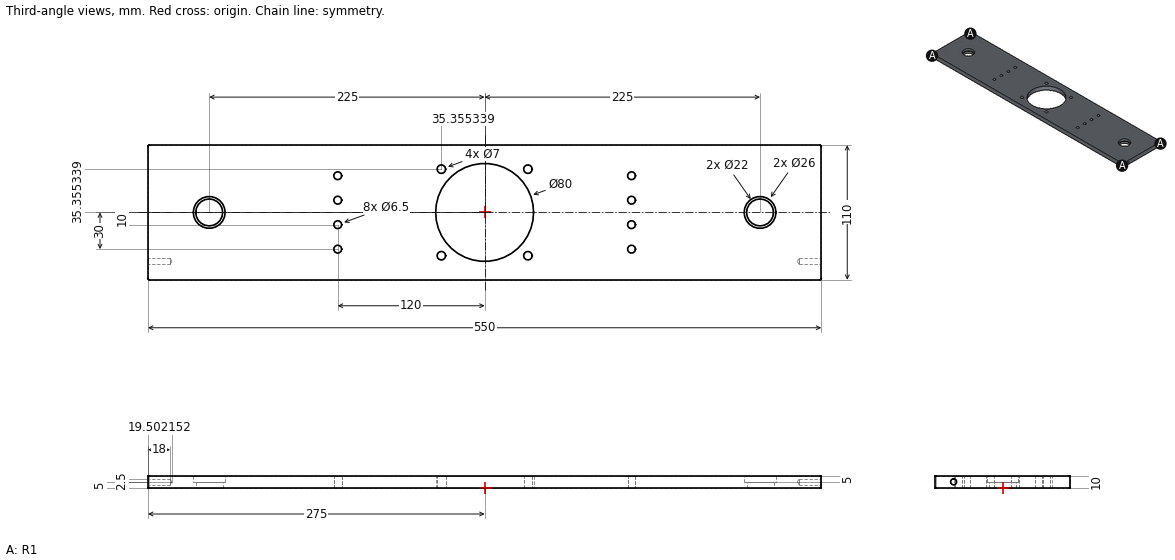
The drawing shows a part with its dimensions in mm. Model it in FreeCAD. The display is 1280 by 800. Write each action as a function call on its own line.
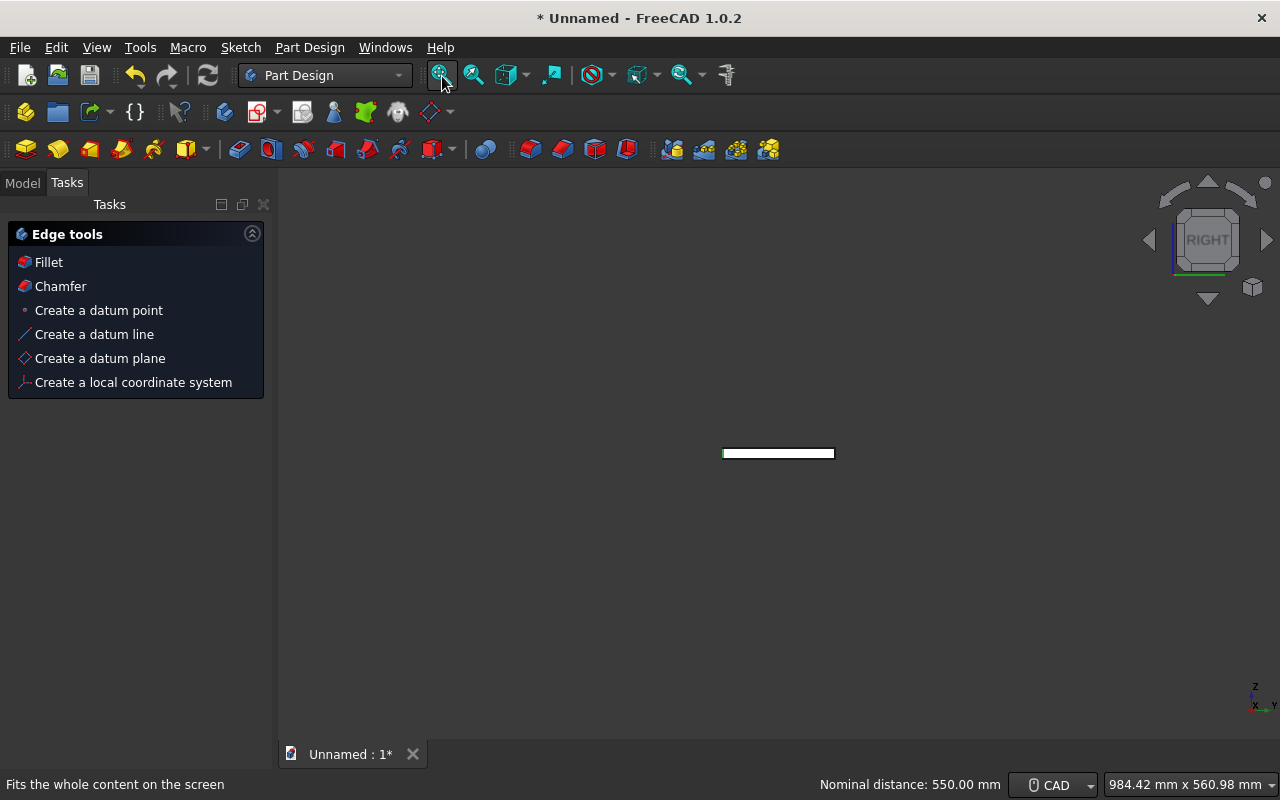
scroll(835, 452, up, 7)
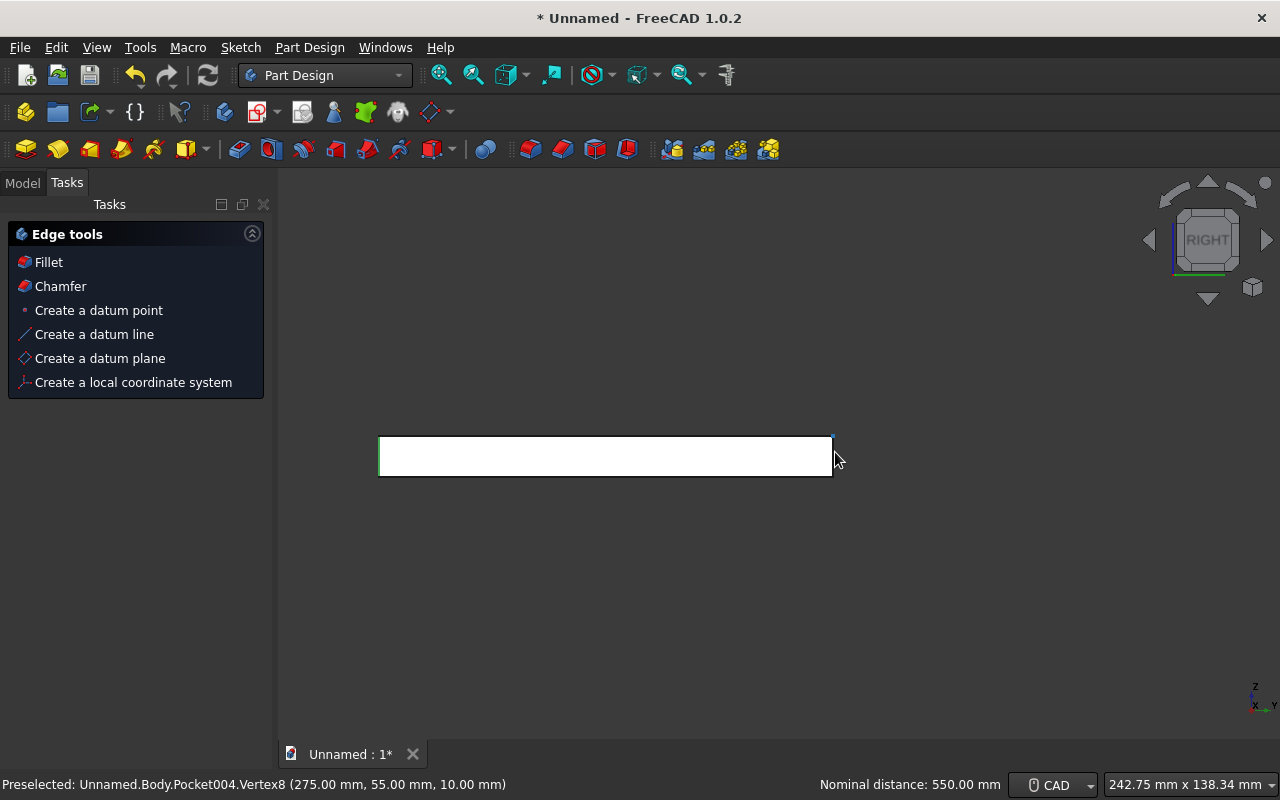
click(833, 456, ctrl)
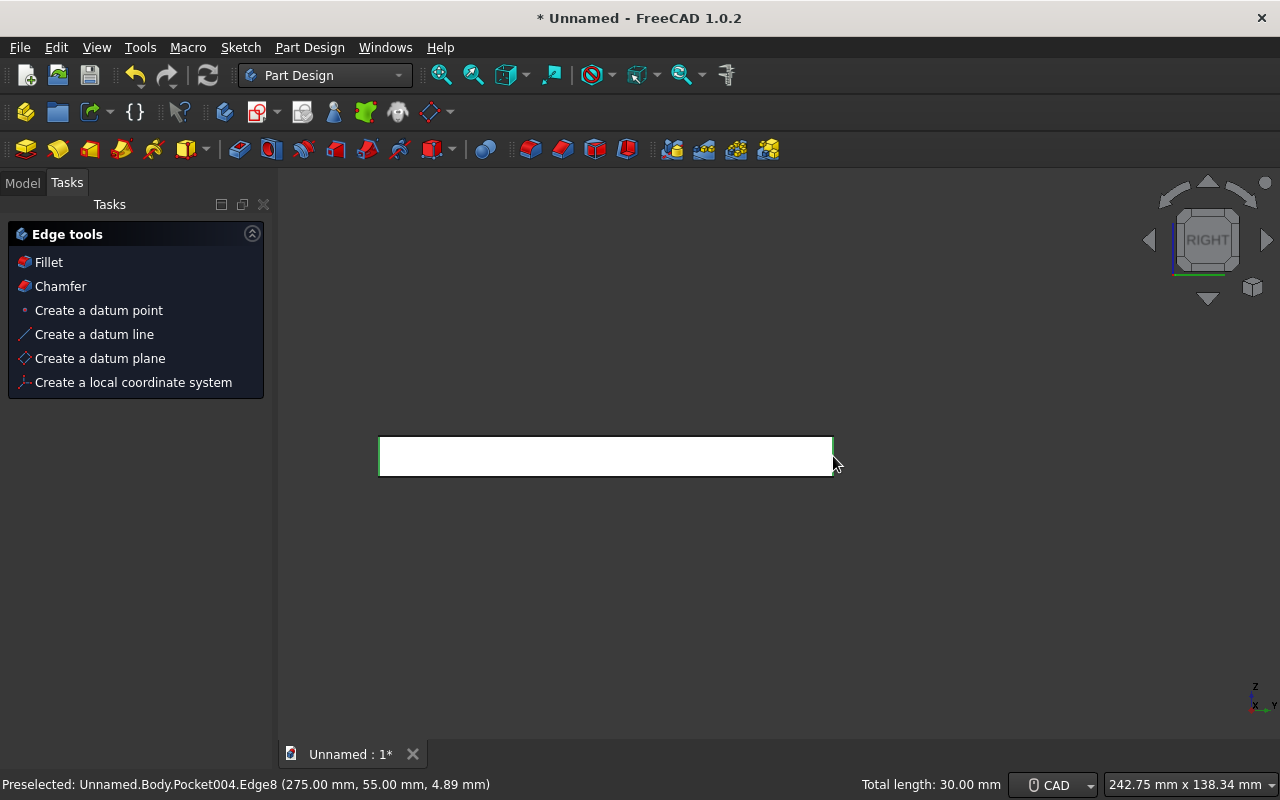
key(v)
key(f)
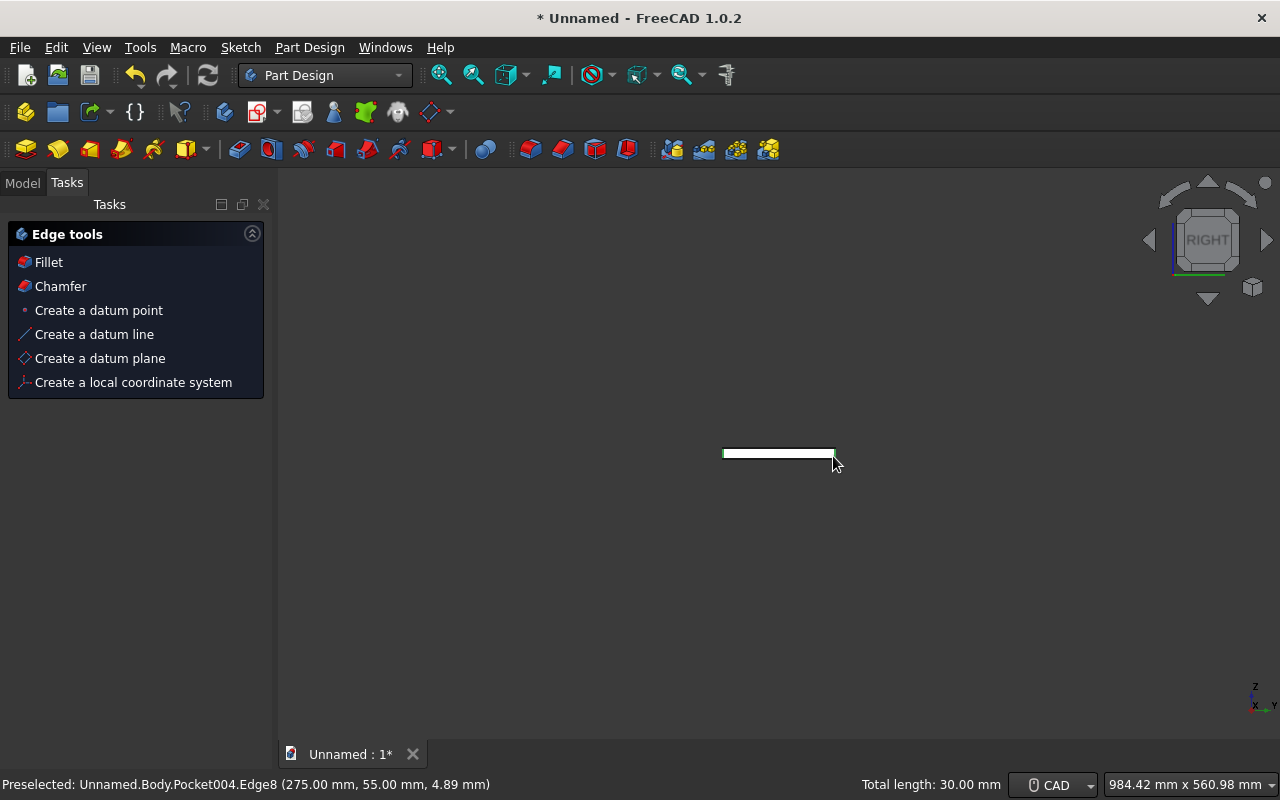
key(5)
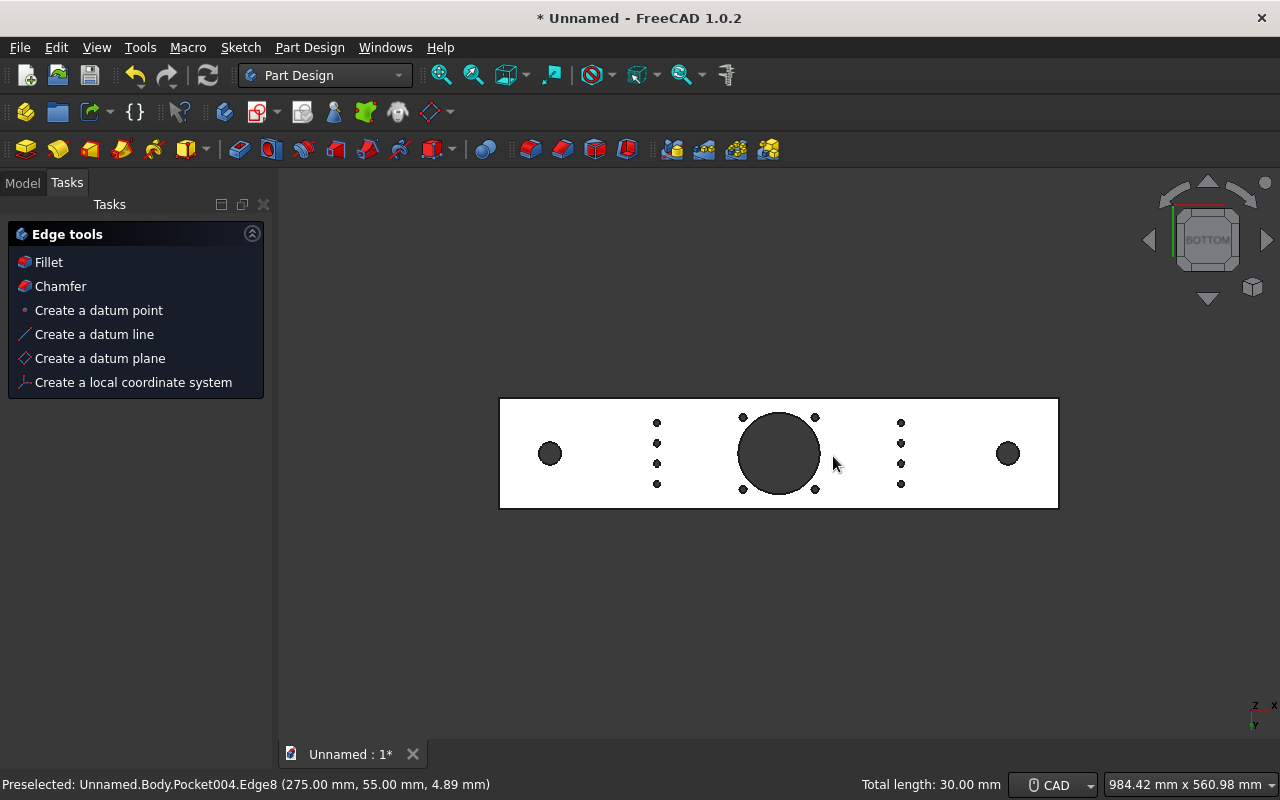
scroll(499, 508, up, 7)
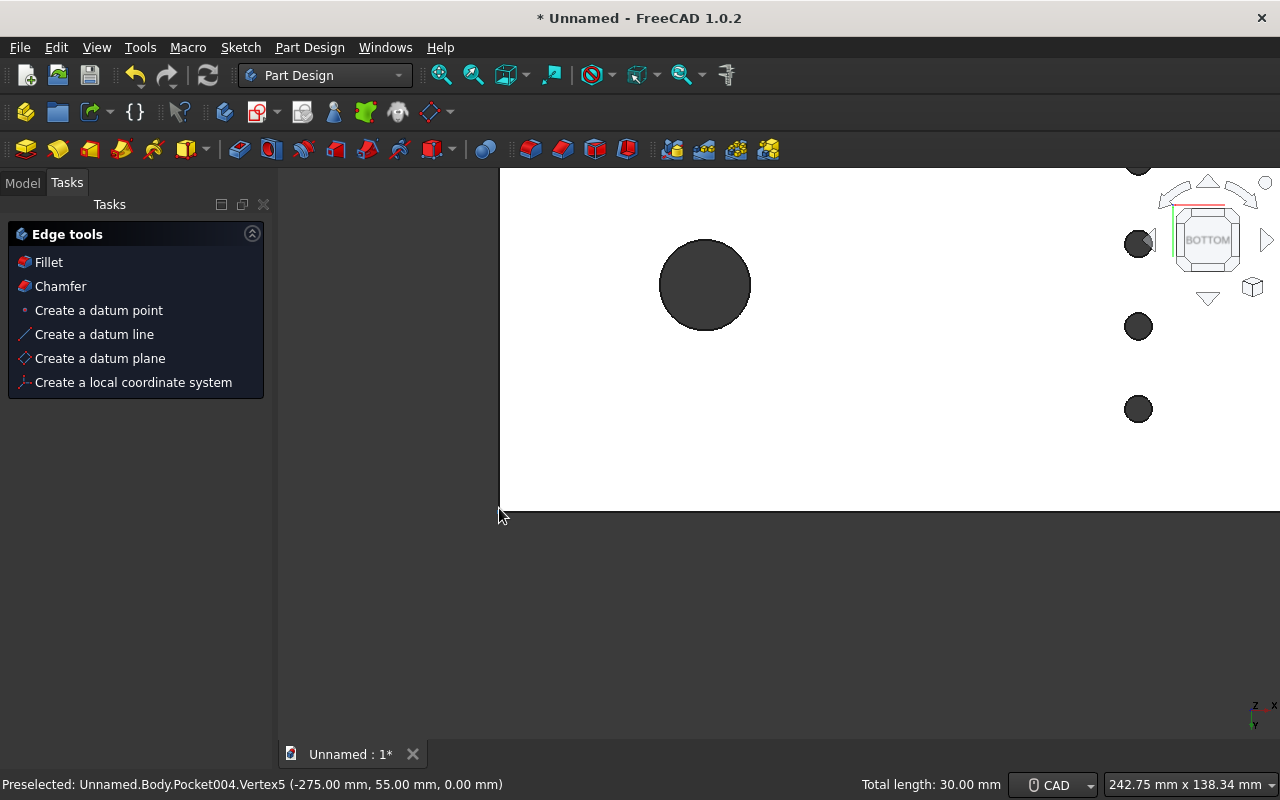
key(v)
key(f)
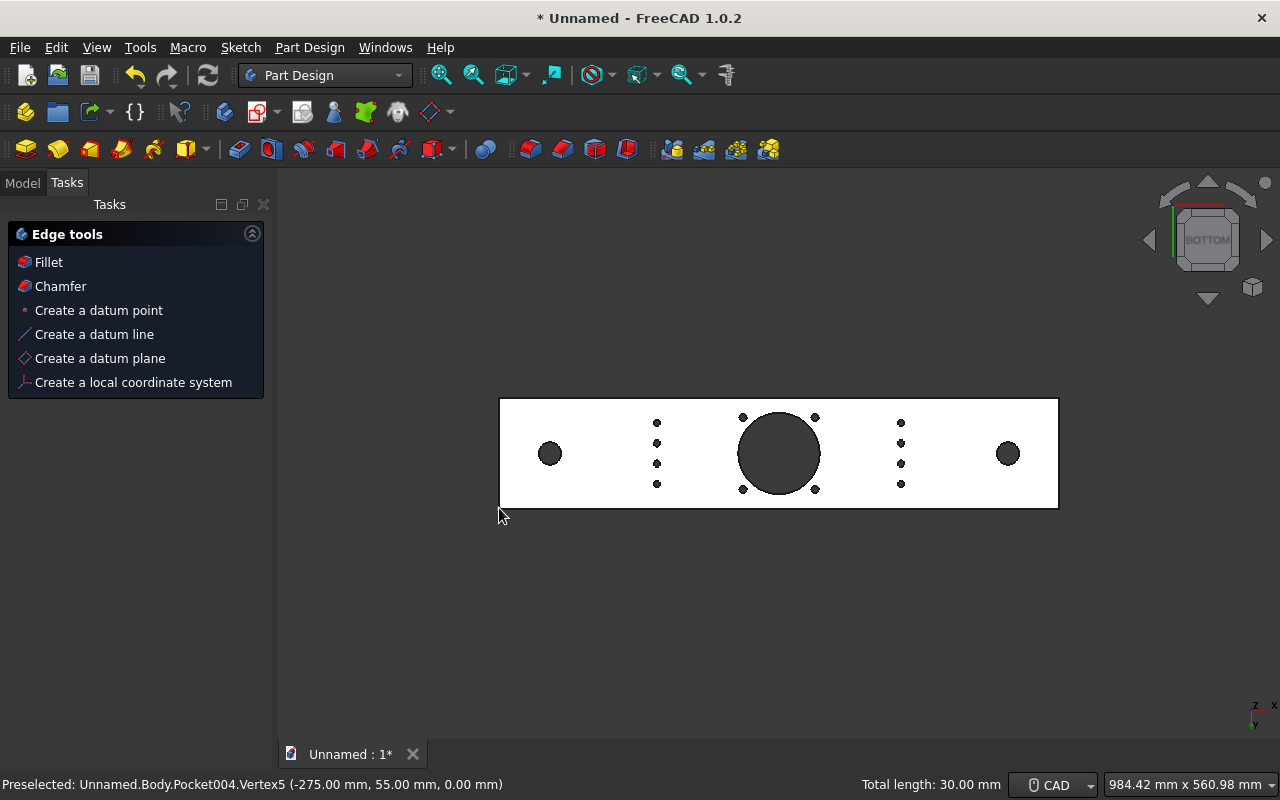
key(4)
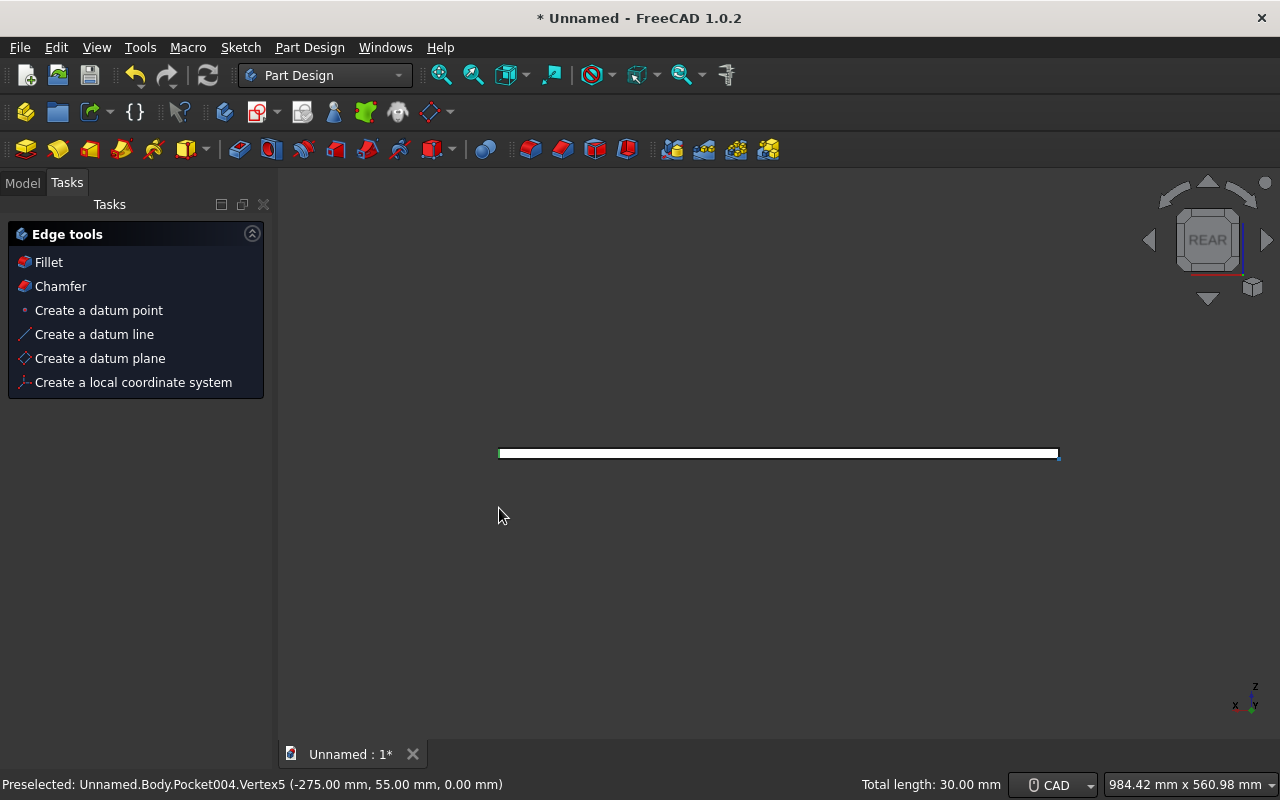
scroll(1059, 452, up, 7)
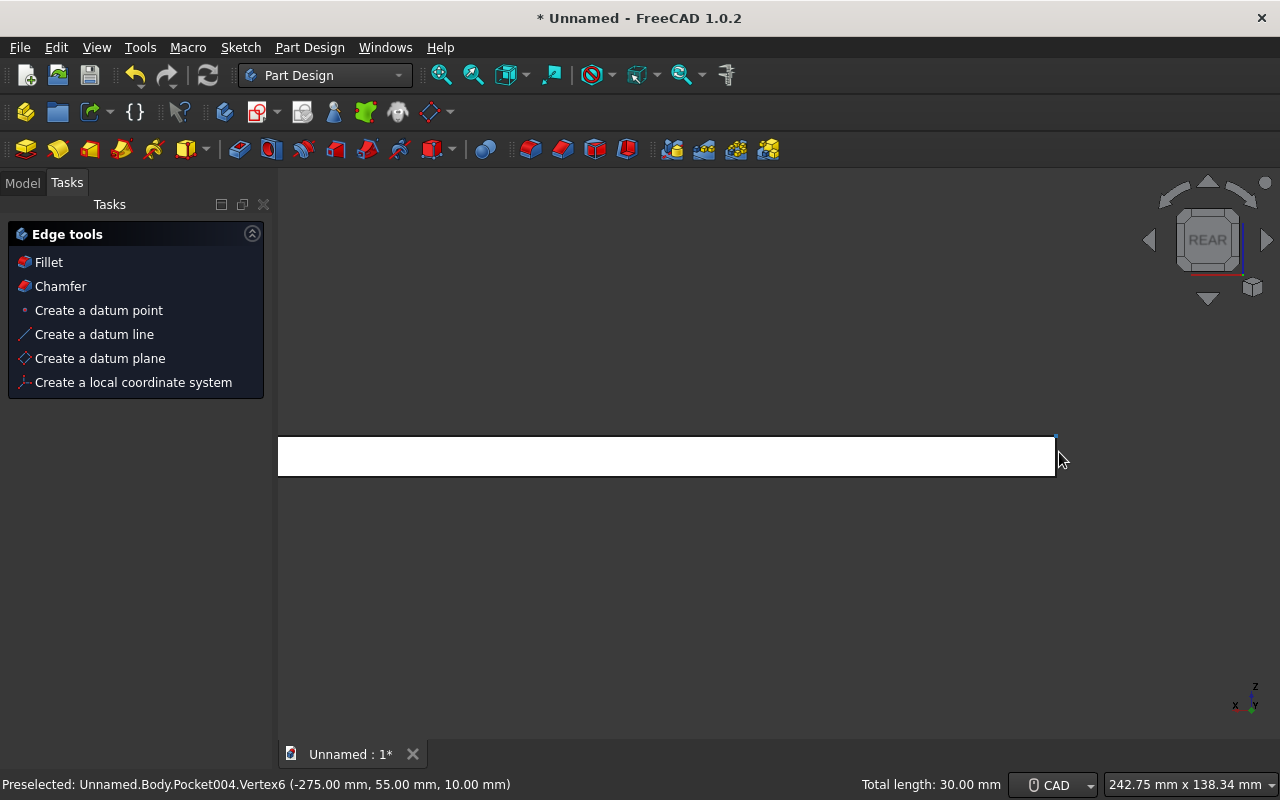
click(1056, 456, ctrl)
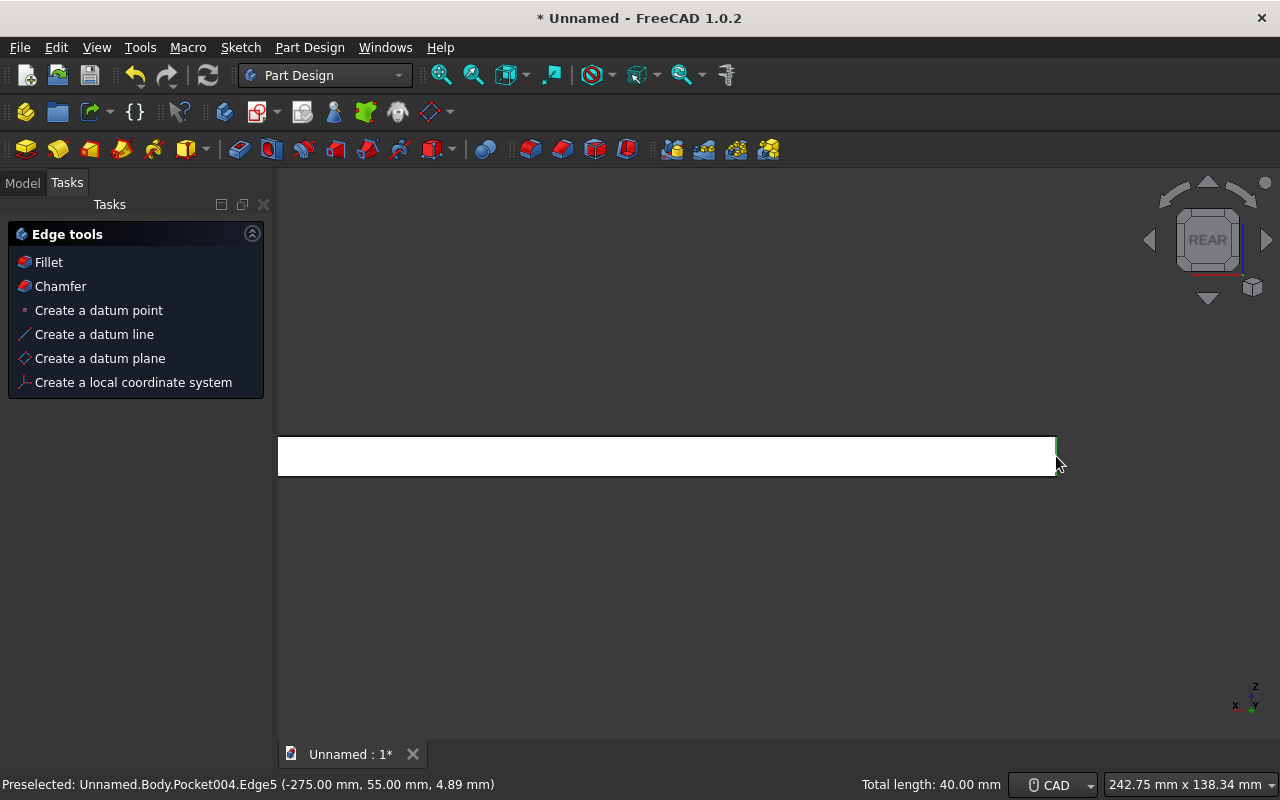
click(532, 150)